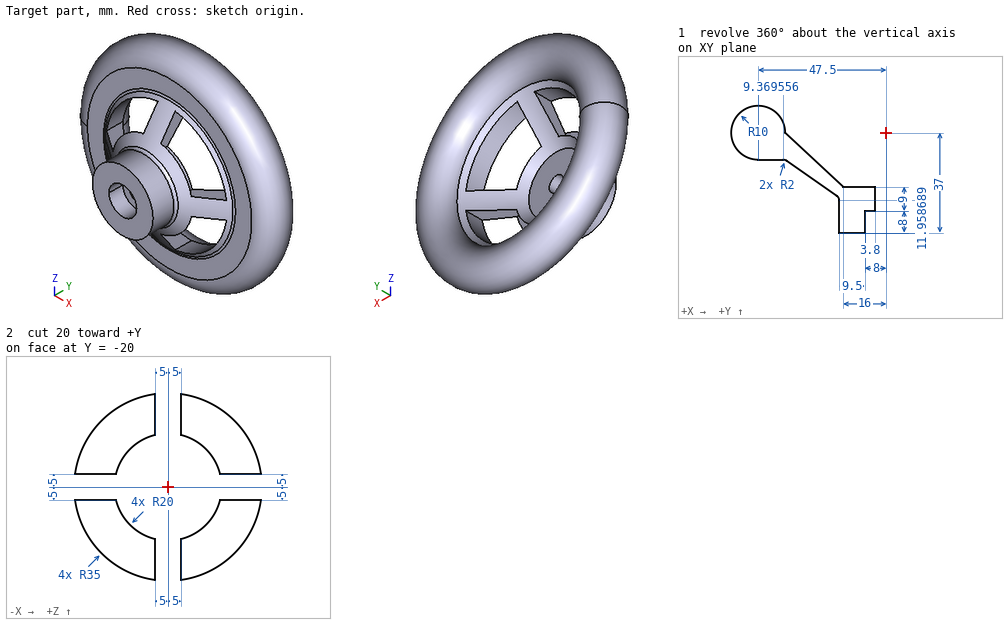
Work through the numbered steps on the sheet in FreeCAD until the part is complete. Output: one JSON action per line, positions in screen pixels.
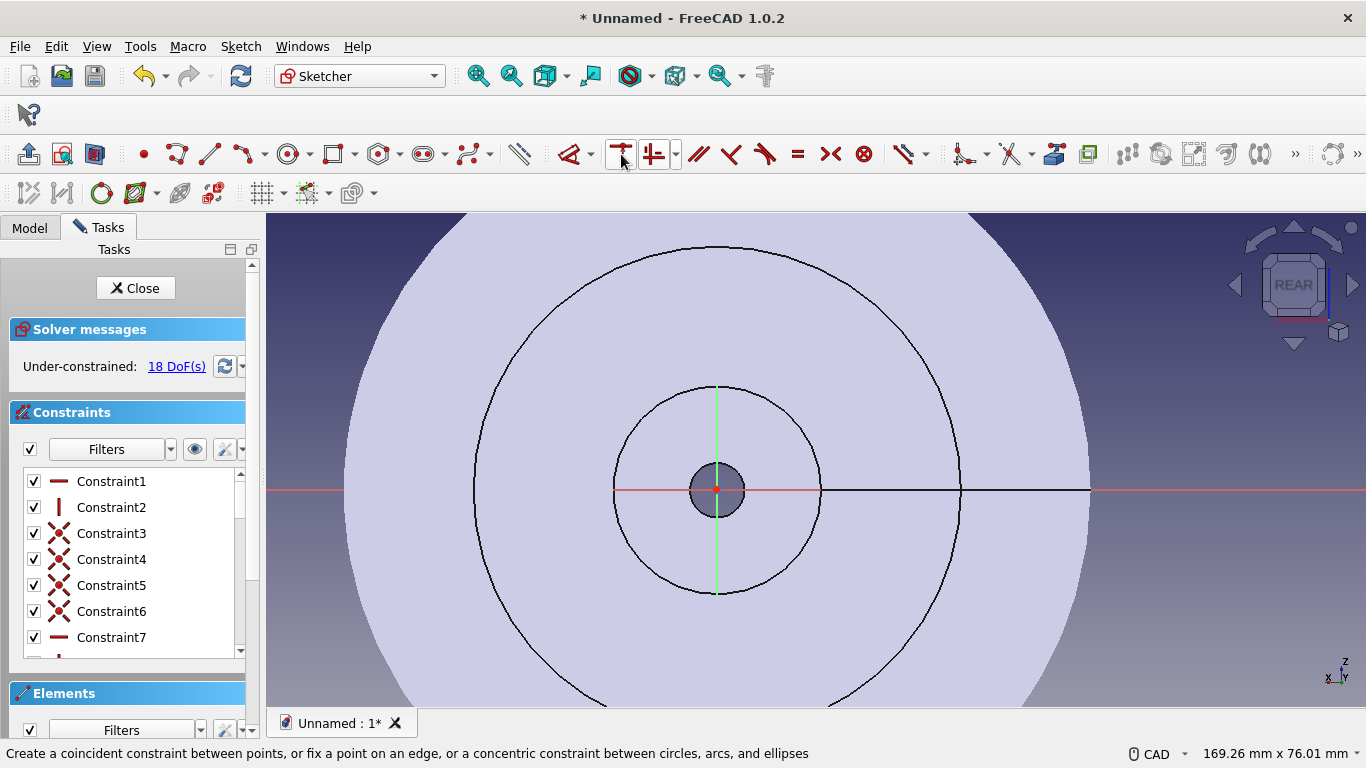
{"action": "left_click_drag", "start_coordinate": [706, 479], "coordinate": [727, 500]}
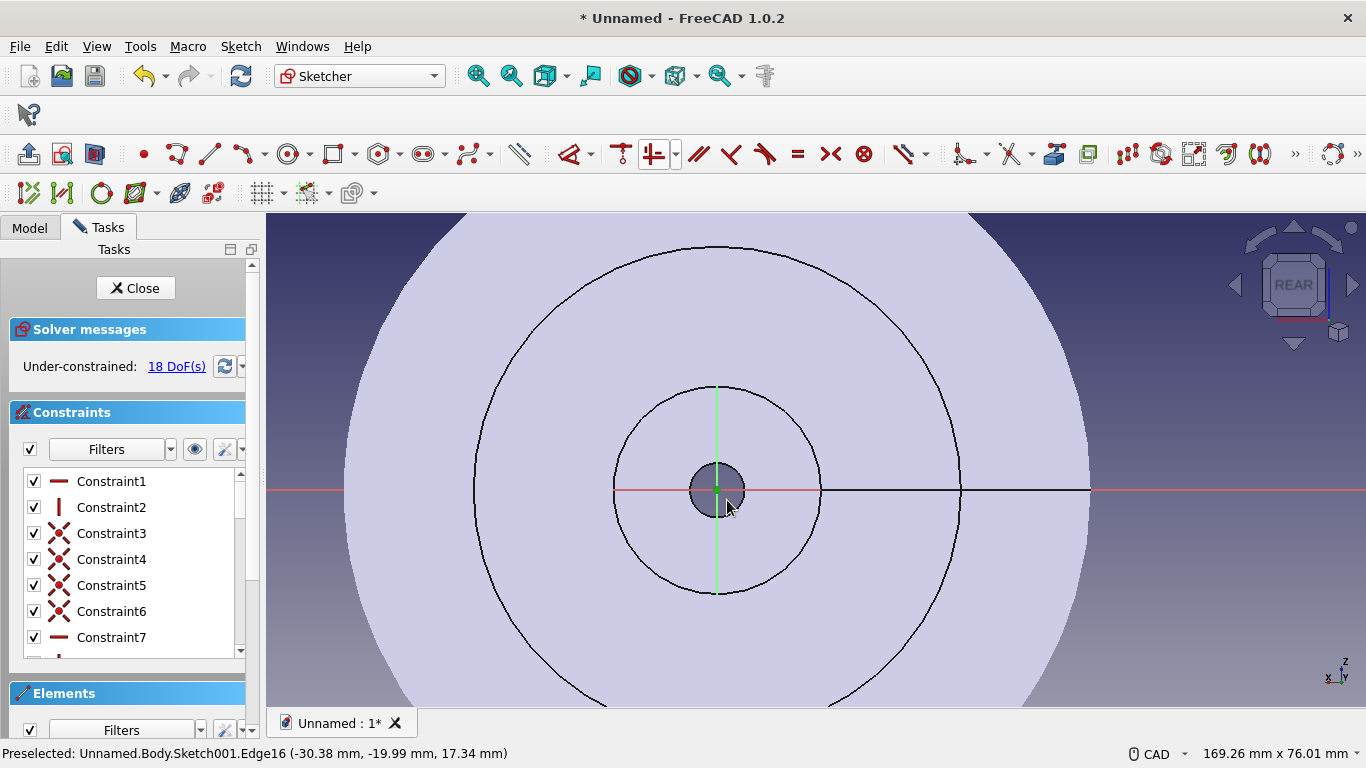
{"action": "left_click", "coordinate": [621, 154]}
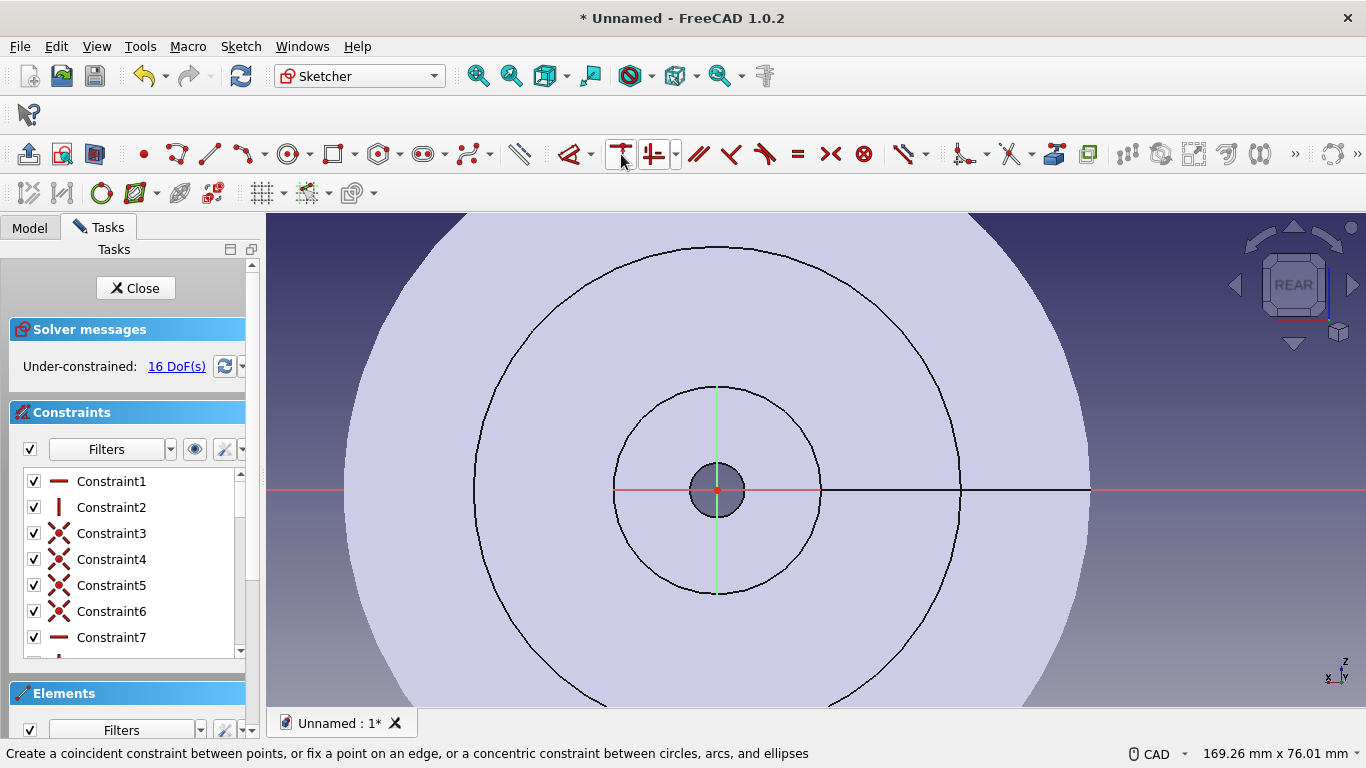
{"action": "left_click", "coordinate": [608, 561]}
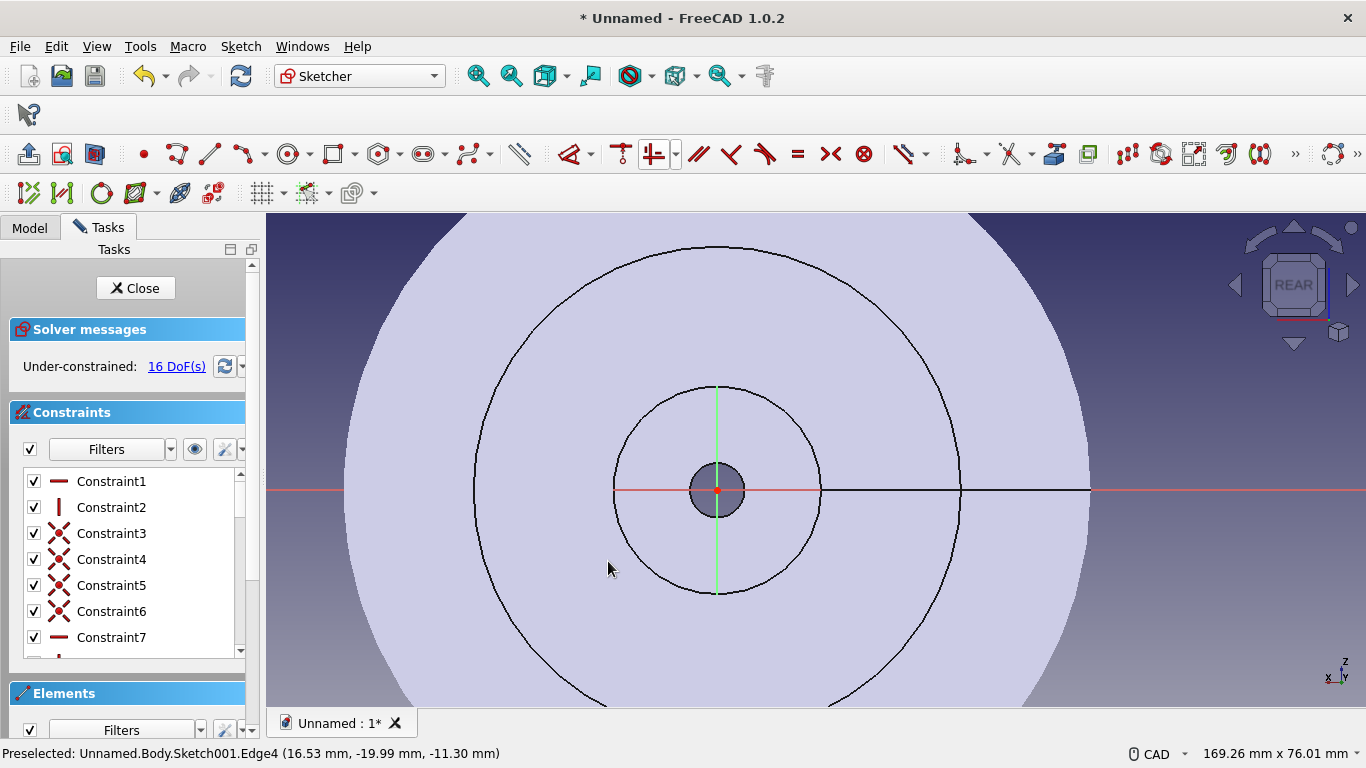
{"action": "left_click", "coordinate": [647, 382]}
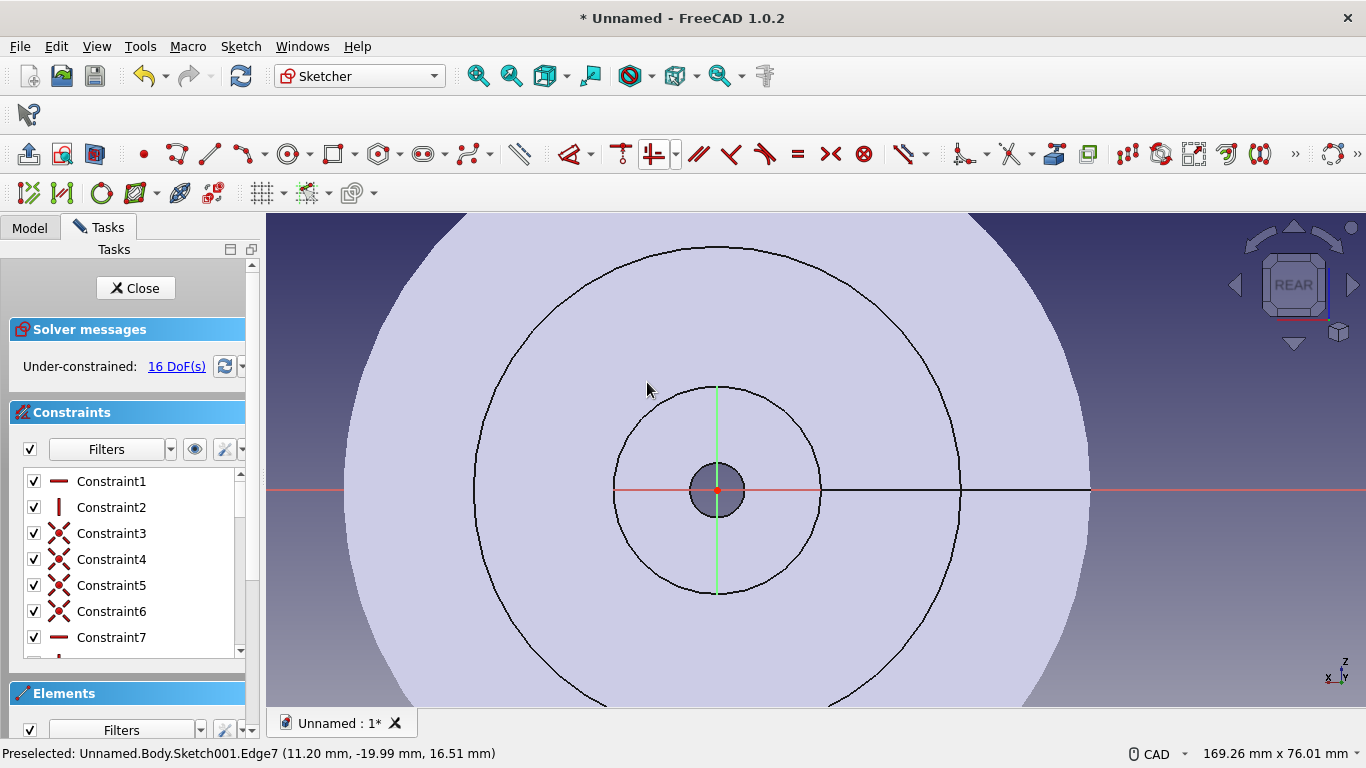
{"action": "left_click", "coordinate": [787, 600]}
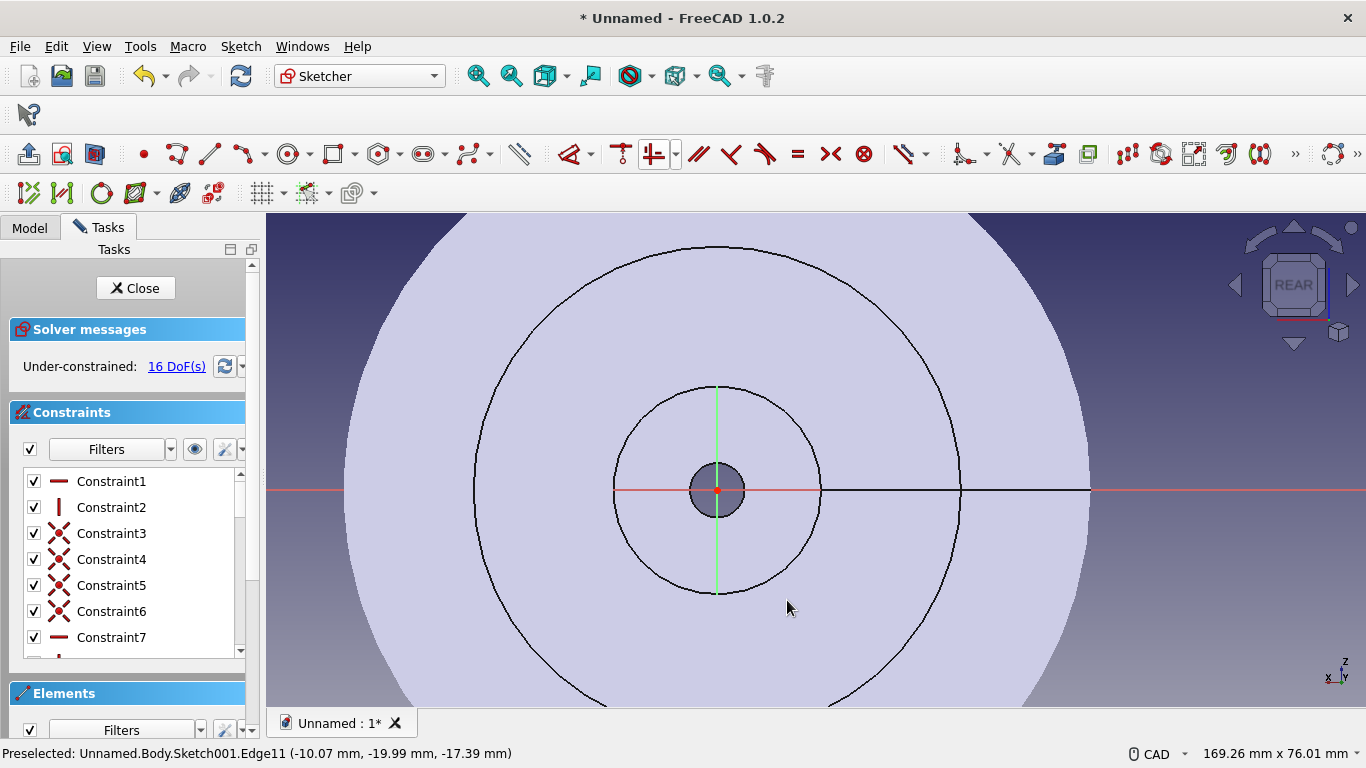
{"action": "left_click", "coordinate": [826, 422]}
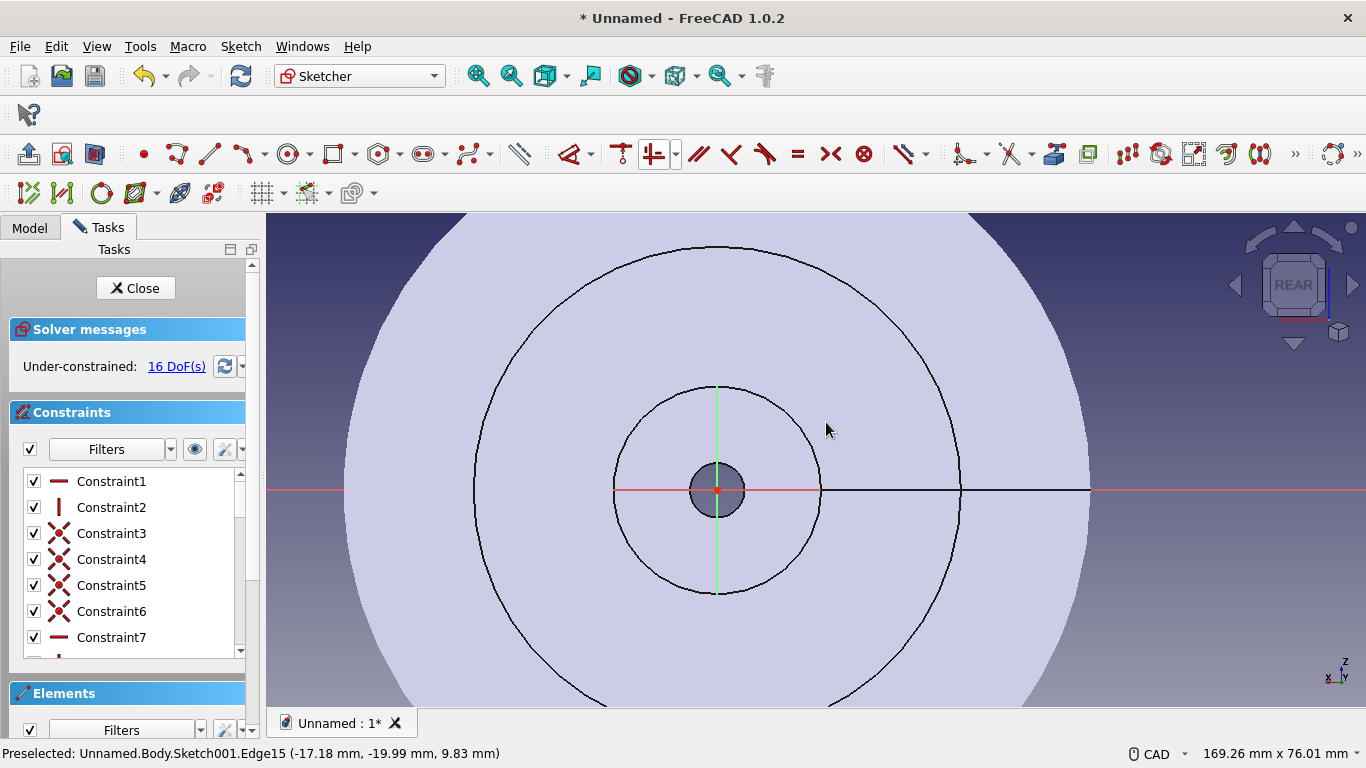
{"action": "left_click", "coordinate": [798, 154]}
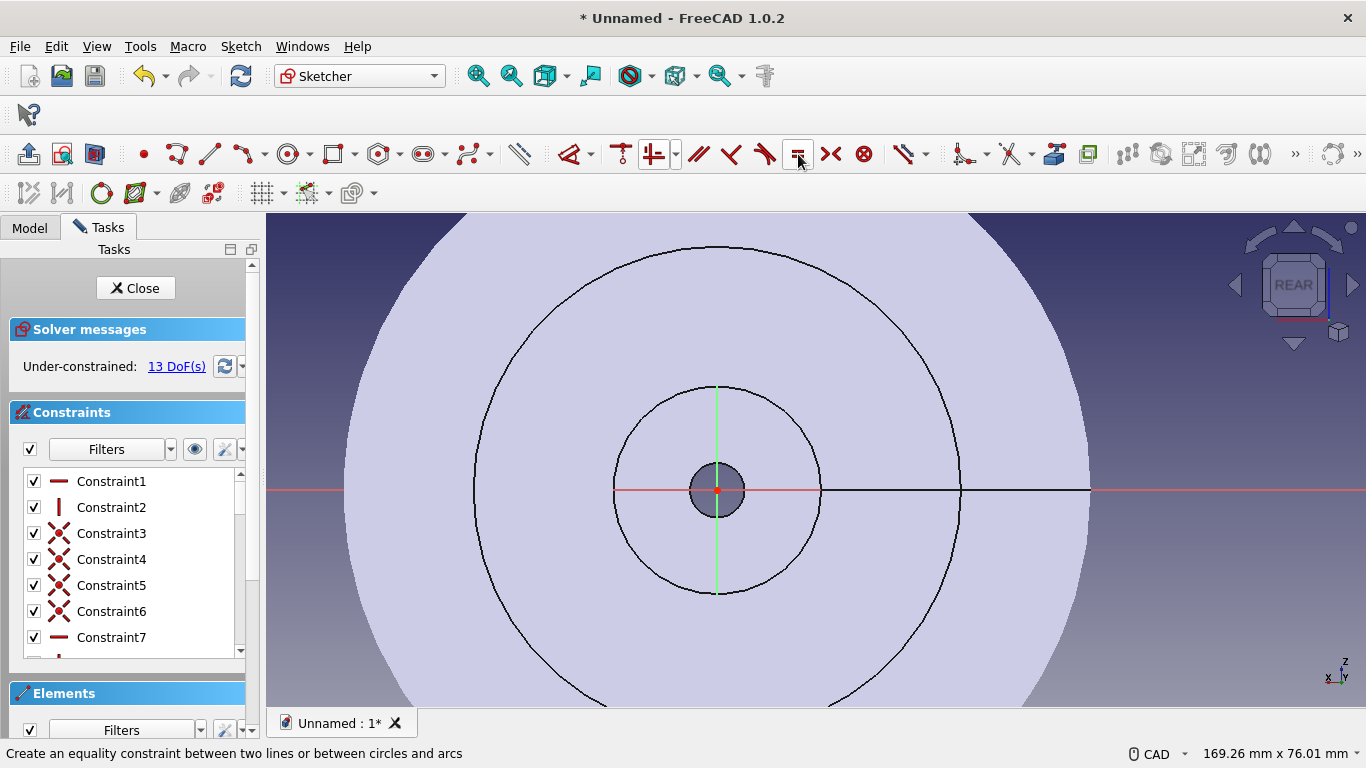
{"action": "left_click", "coordinate": [521, 606]}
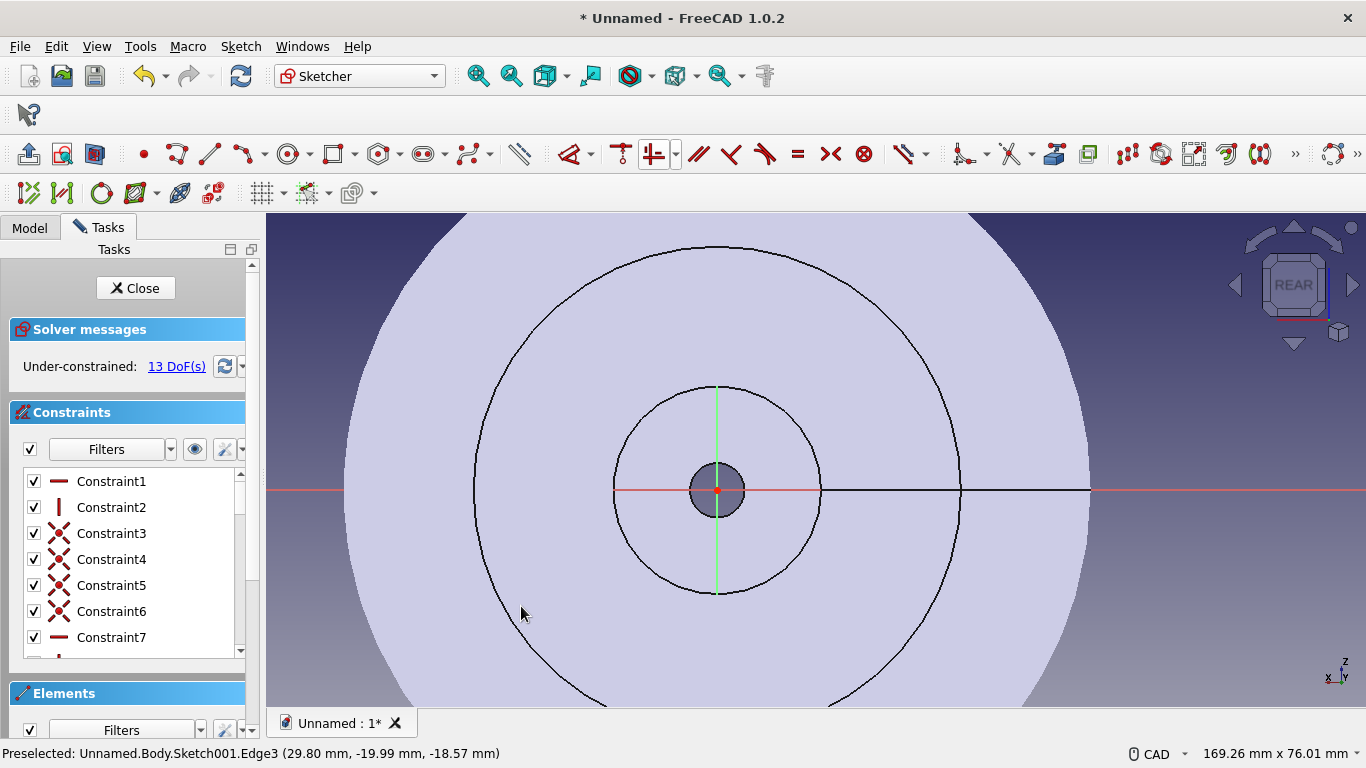
{"action": "left_click", "coordinate": [603, 295]}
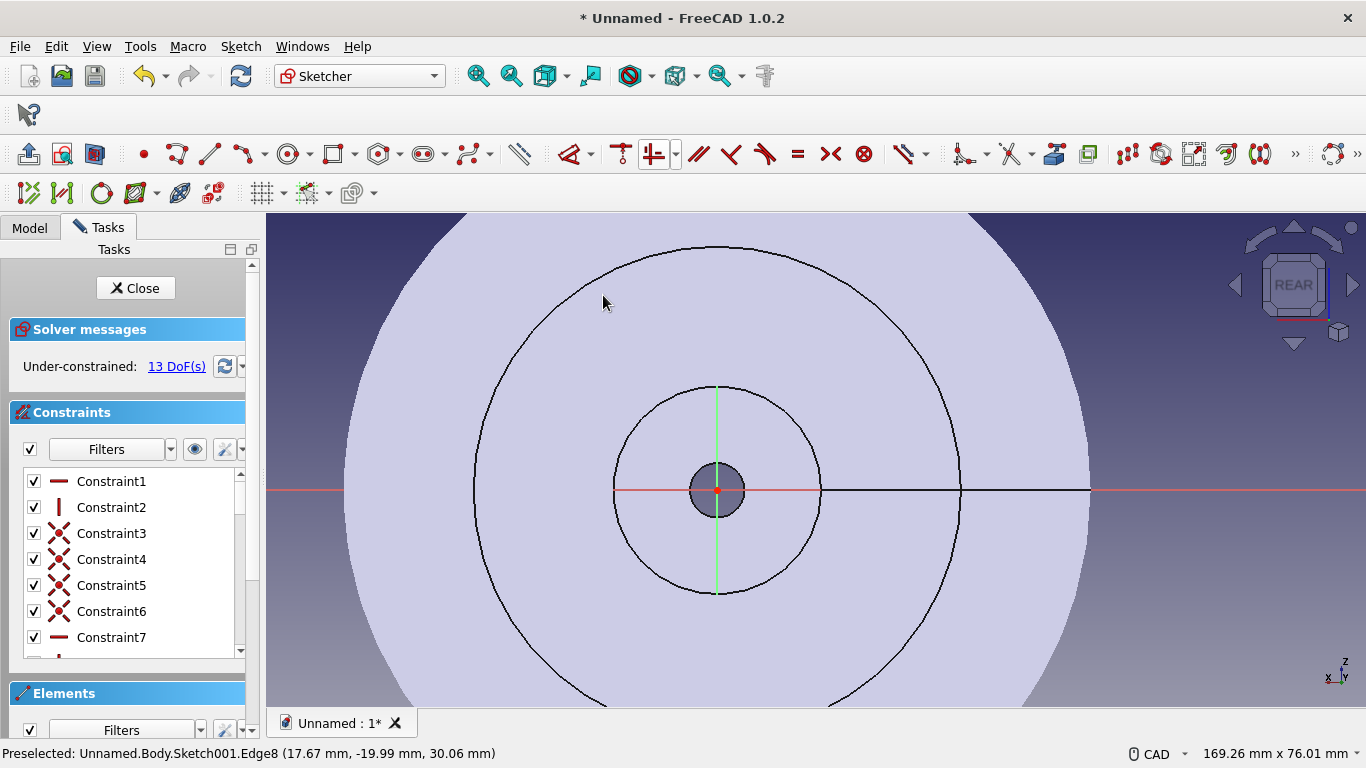
{"action": "left_click", "coordinate": [914, 606]}